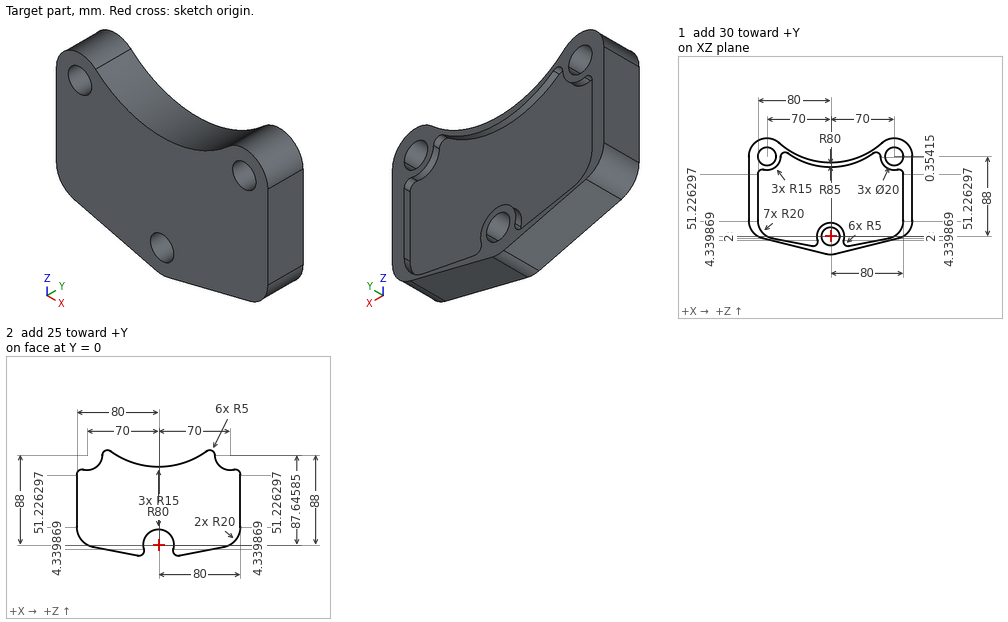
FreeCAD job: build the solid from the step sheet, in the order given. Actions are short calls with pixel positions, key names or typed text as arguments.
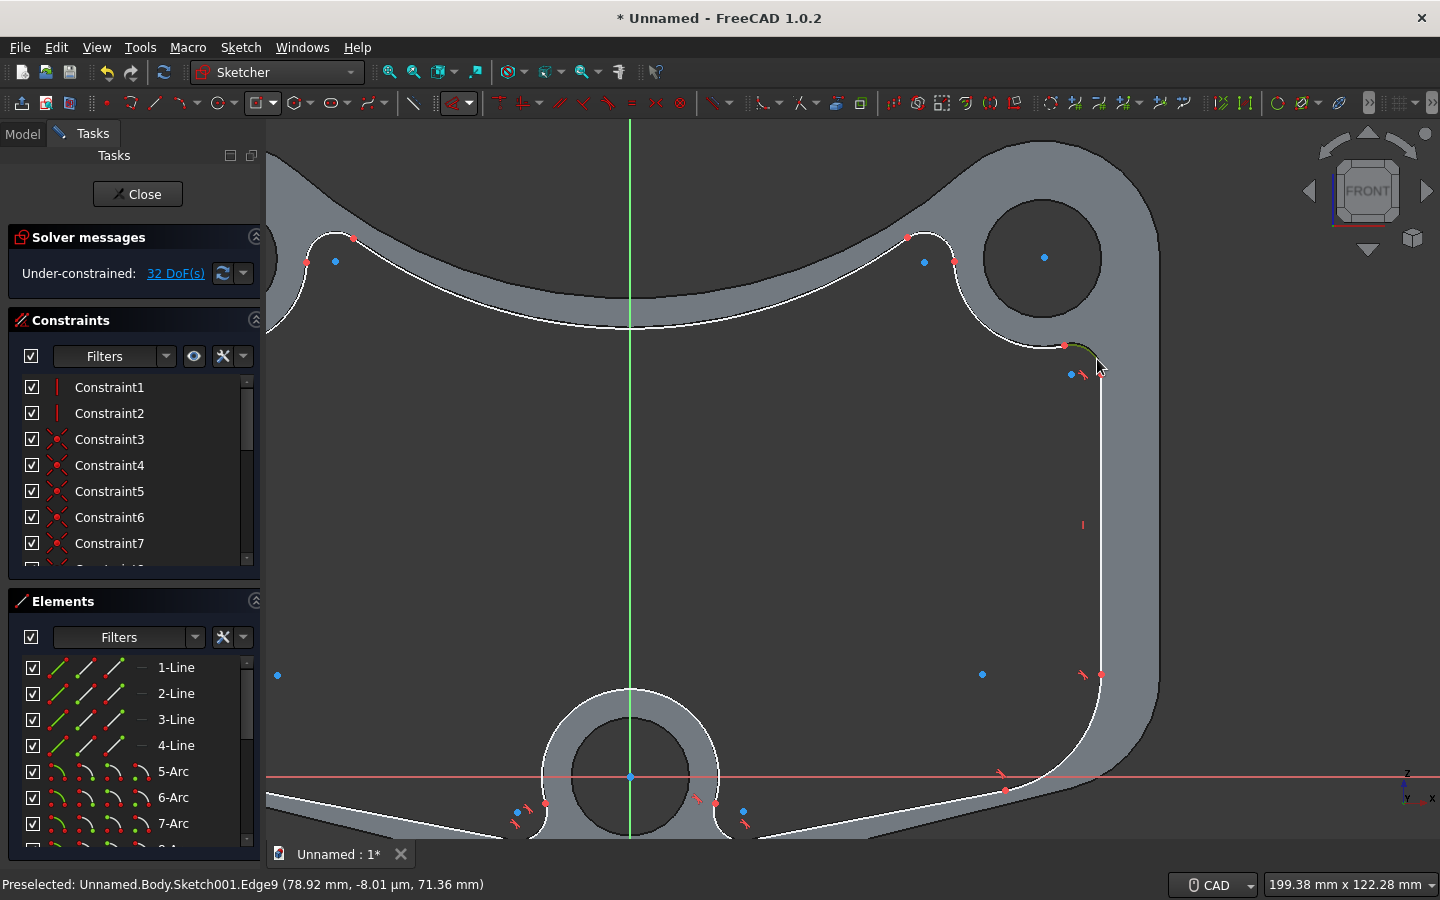
click(968, 306)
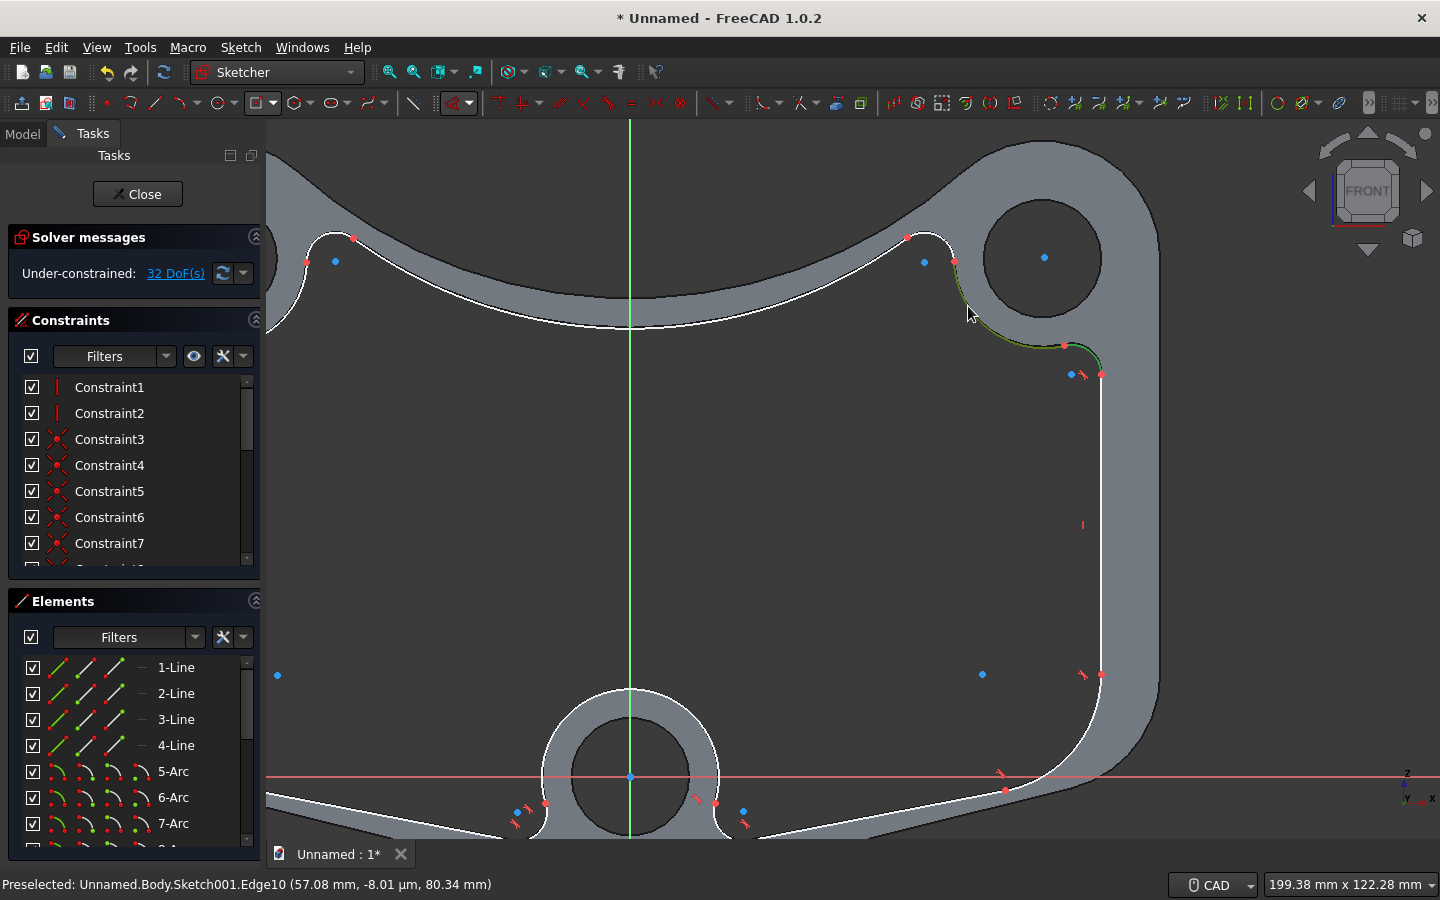
key(t)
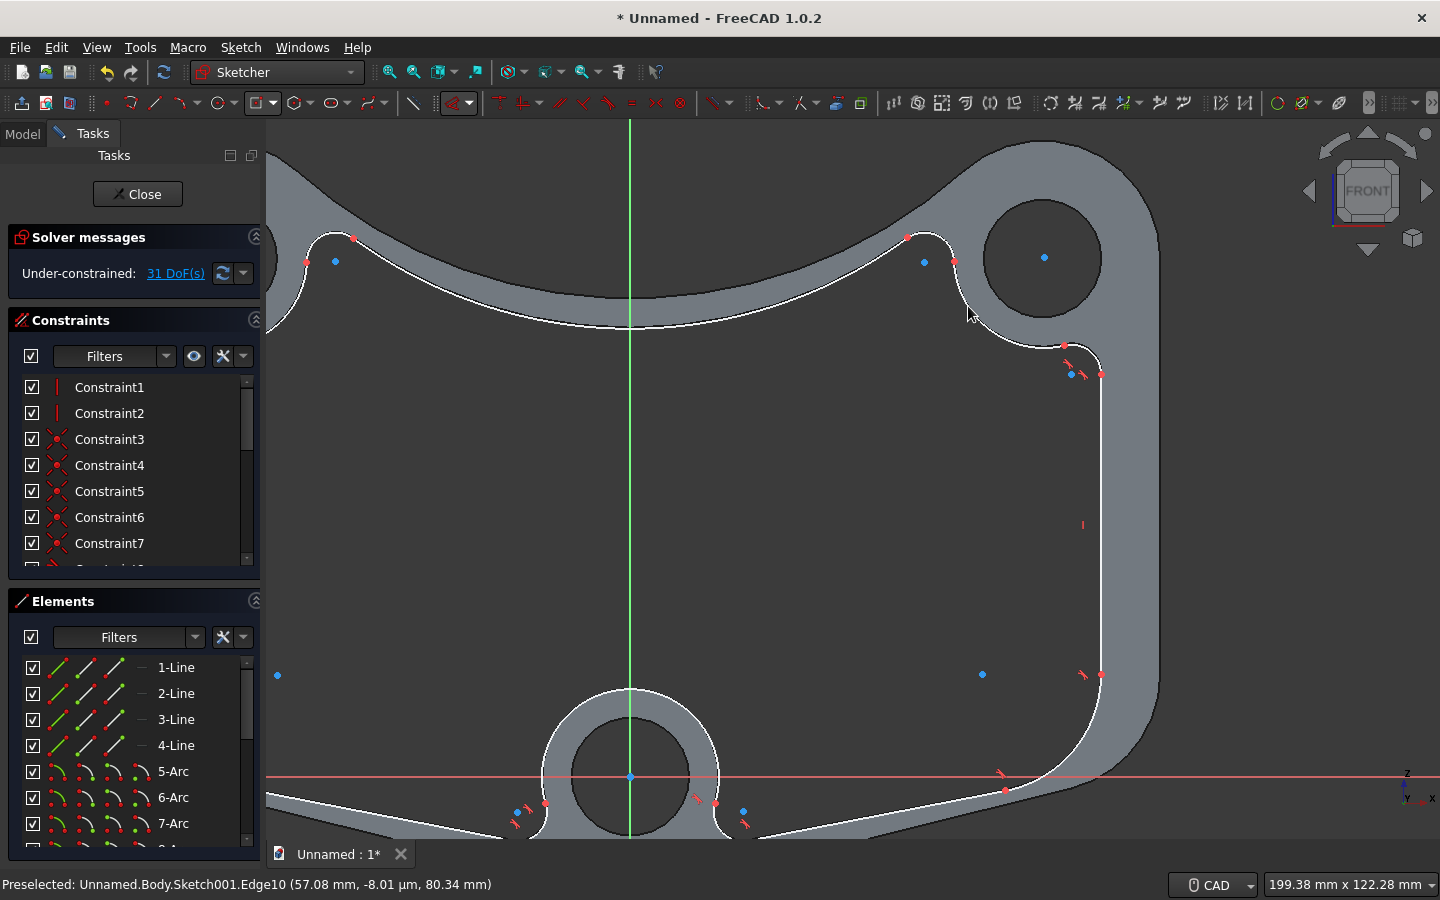
click(968, 306)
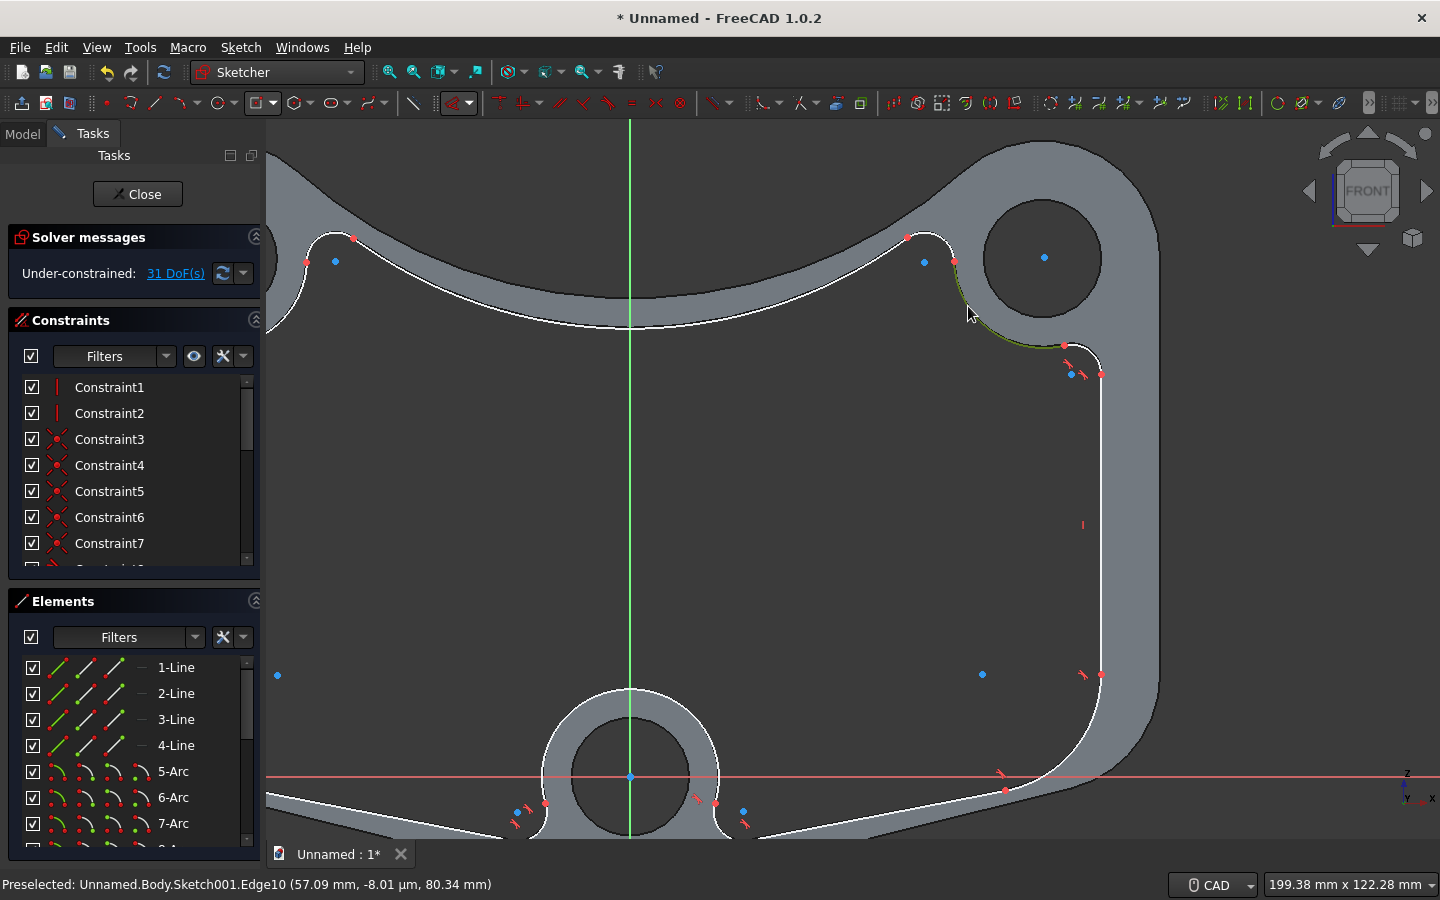
click(948, 244)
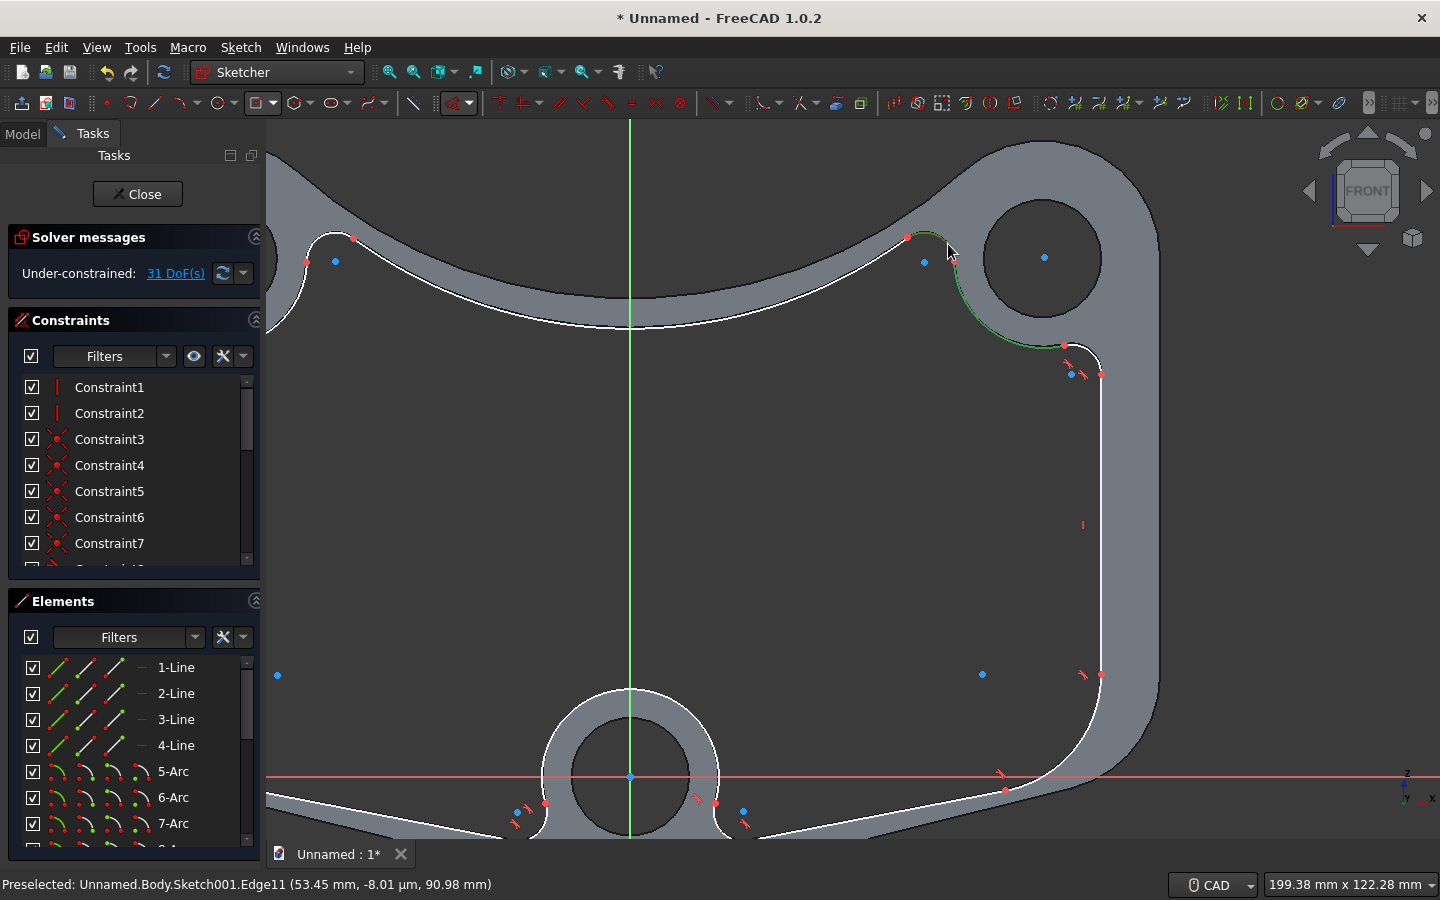
click(608, 104)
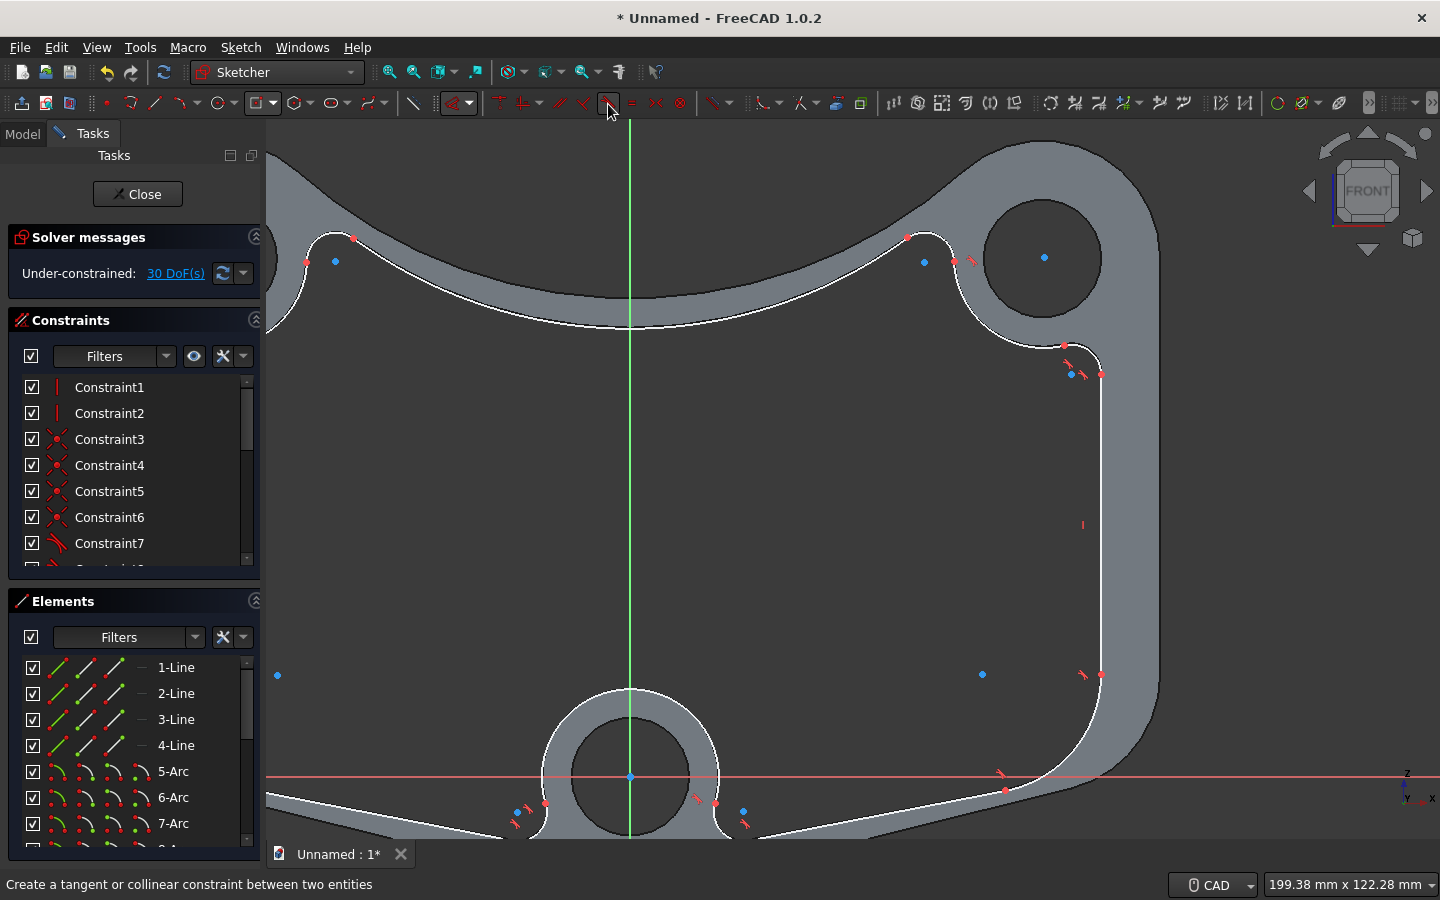
click(948, 244)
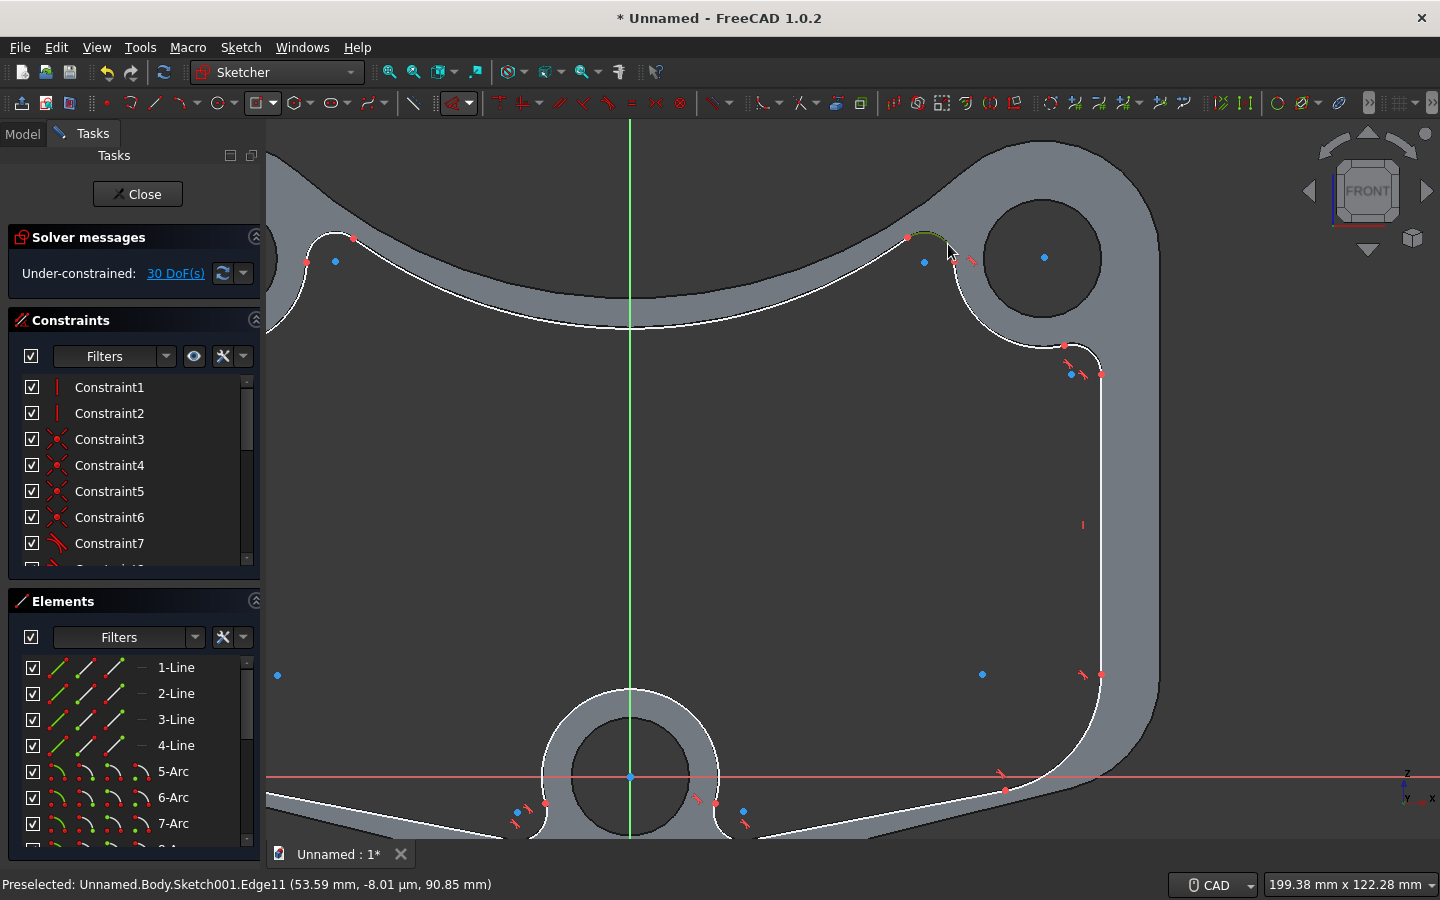
click(513, 314)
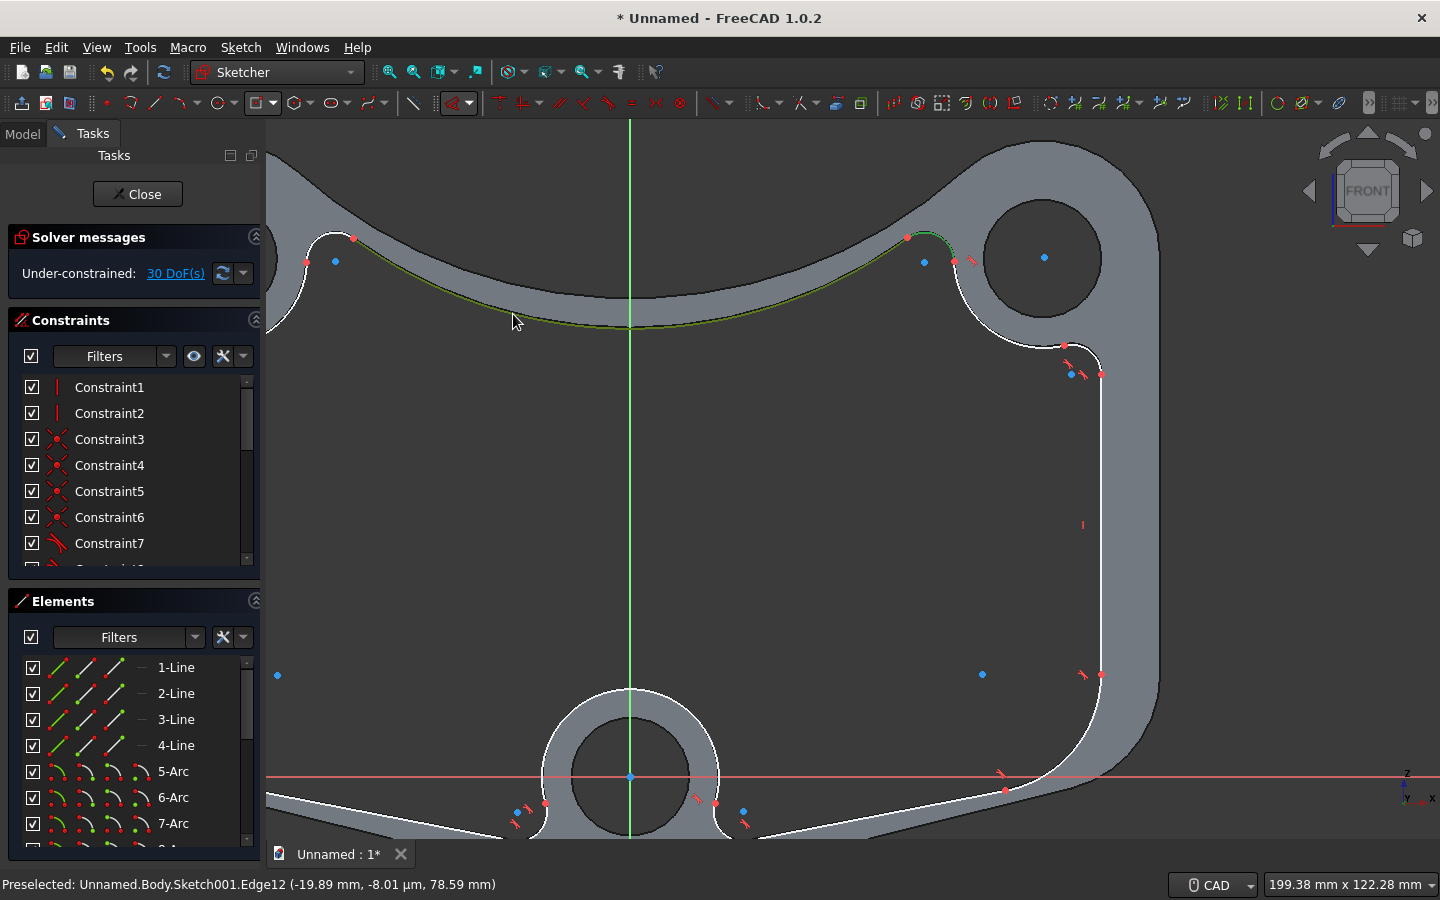
click(608, 104)